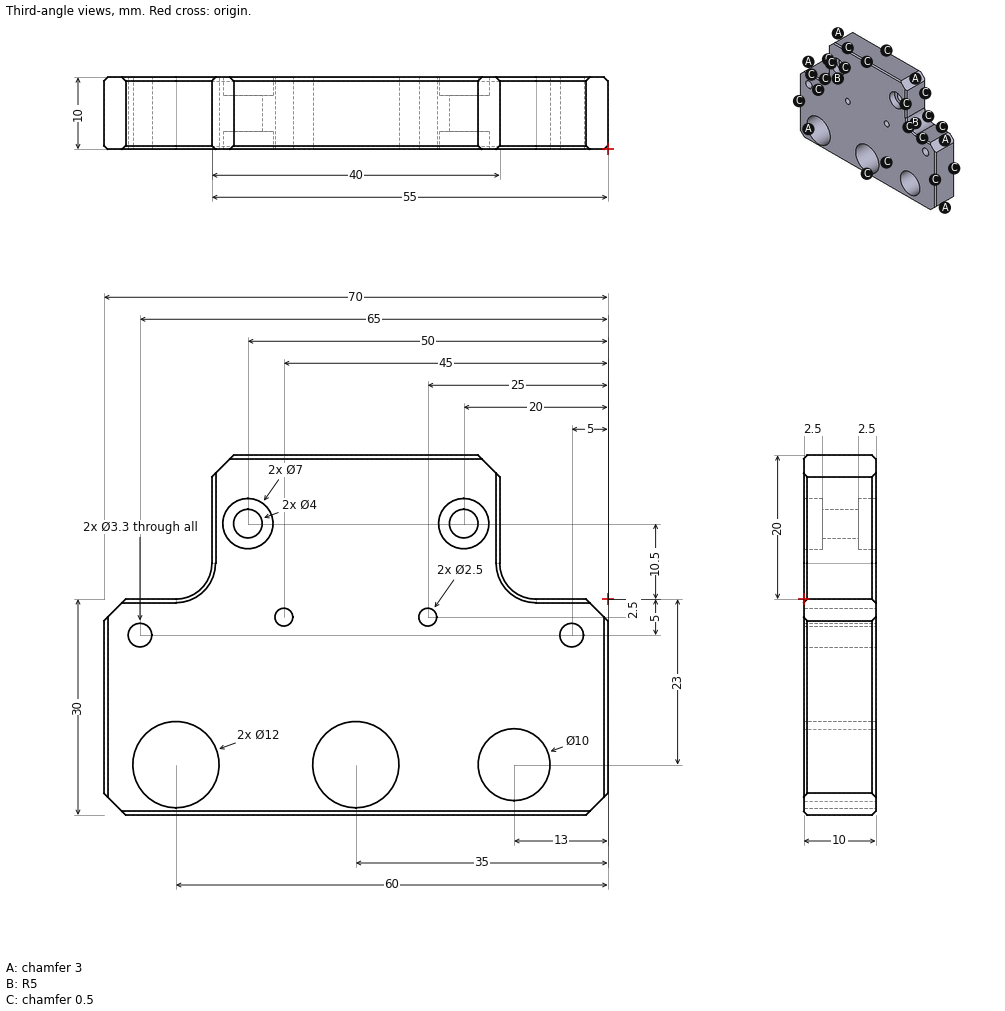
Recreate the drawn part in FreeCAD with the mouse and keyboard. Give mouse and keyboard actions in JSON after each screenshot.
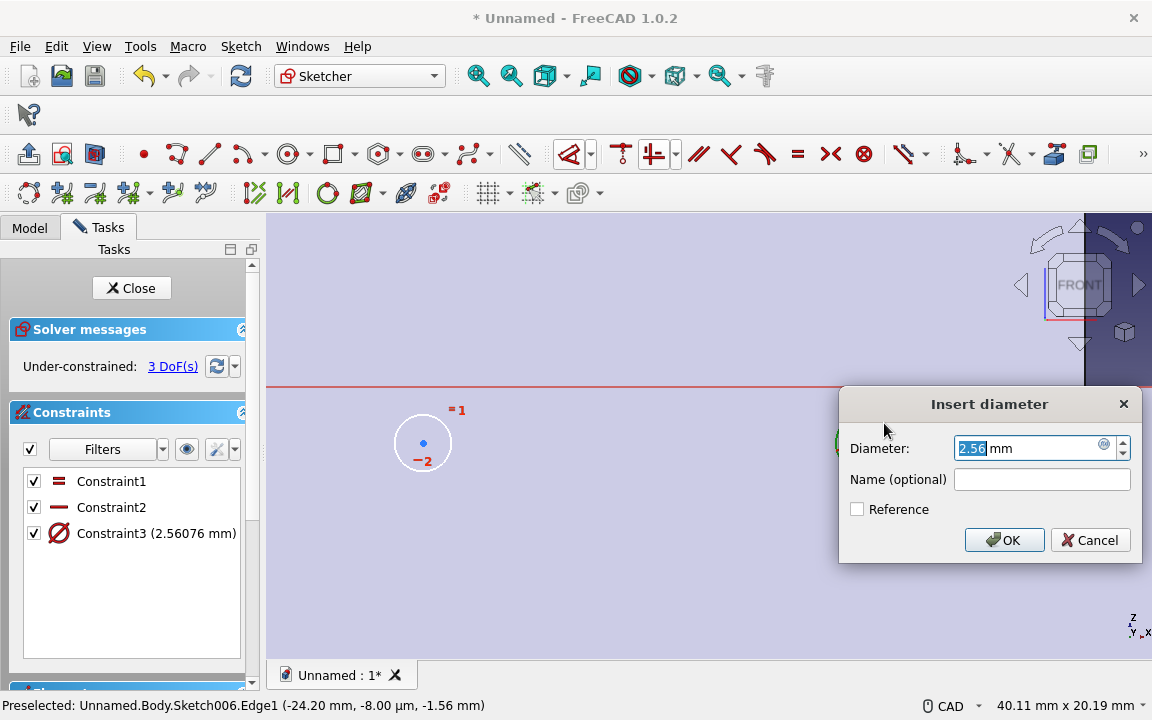
{"action": "type", "text": "2.5"}
{"action": "key", "text": "Return"}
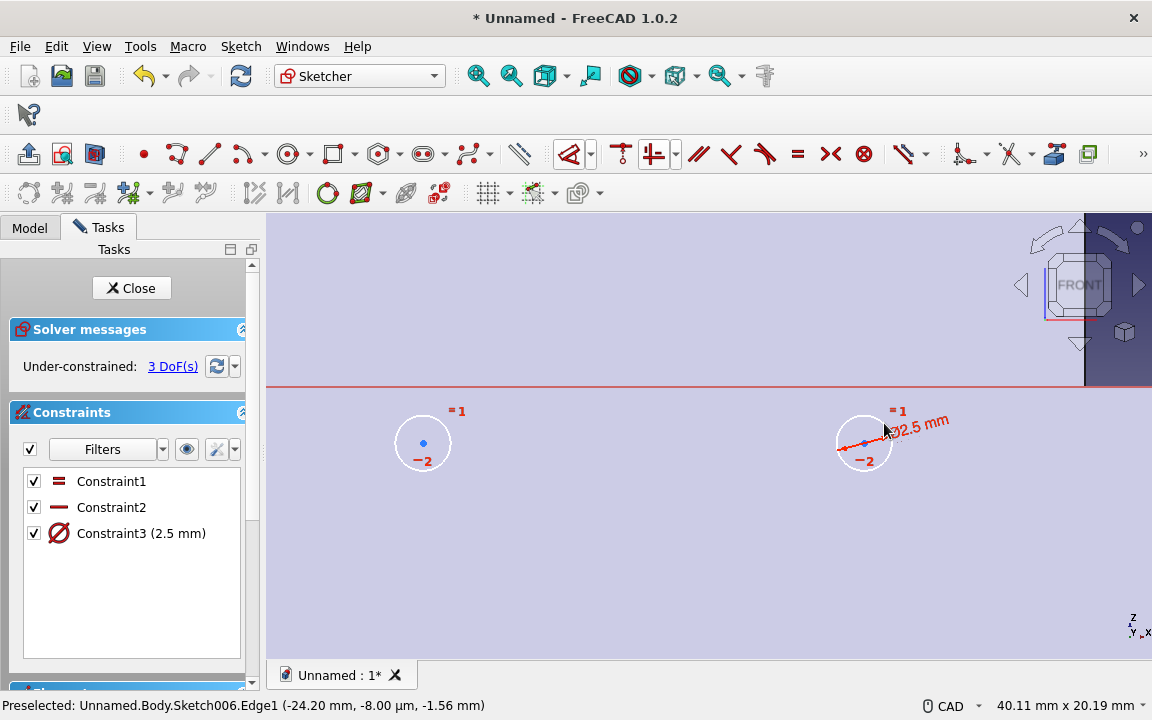
{"action": "left_click", "coordinate": [864, 443]}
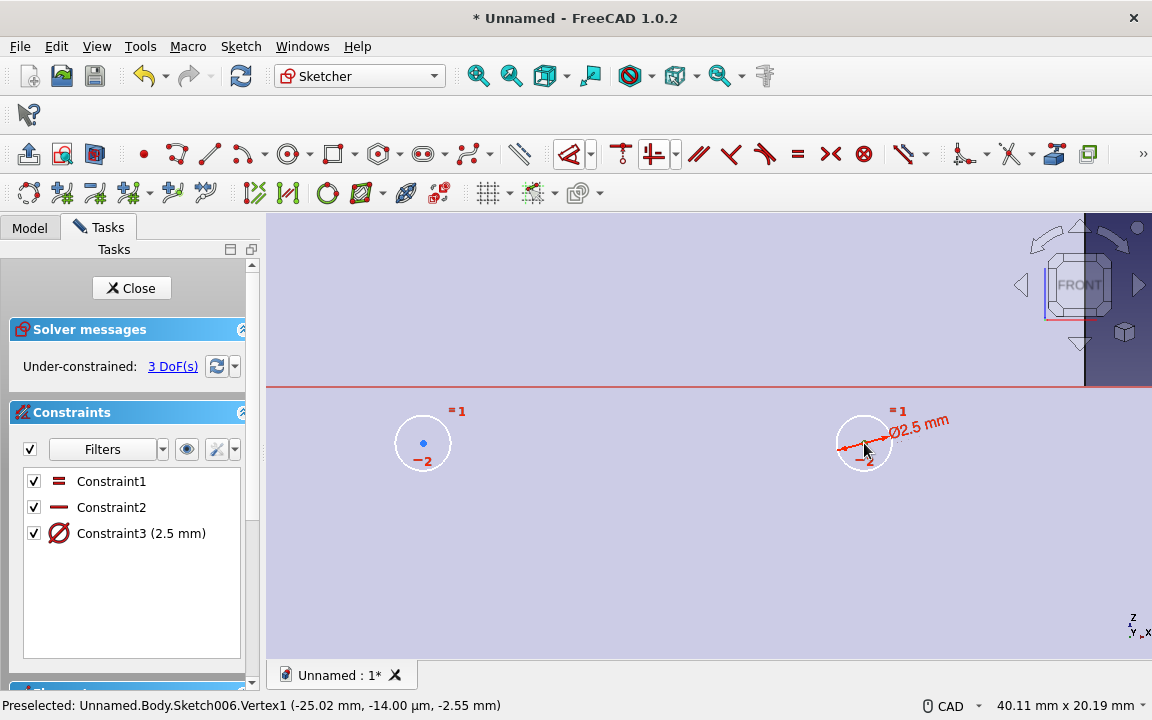
{"action": "left_click", "coordinate": [590, 154]}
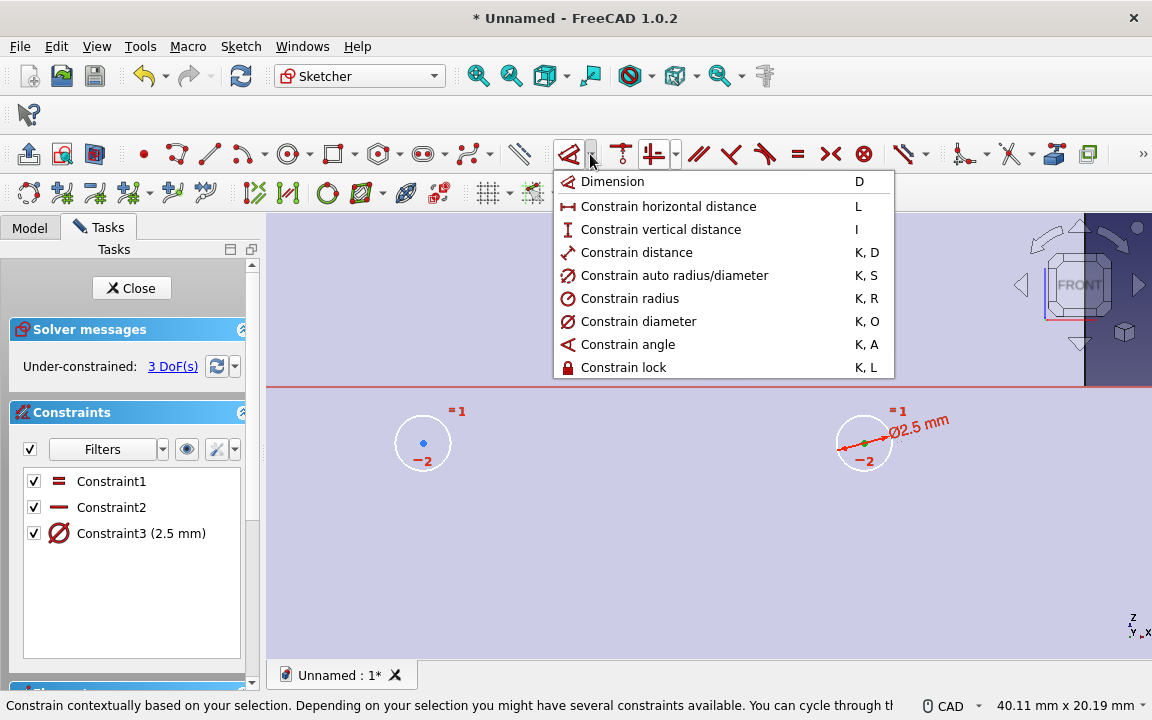
{"action": "left_click", "coordinate": [724, 206]}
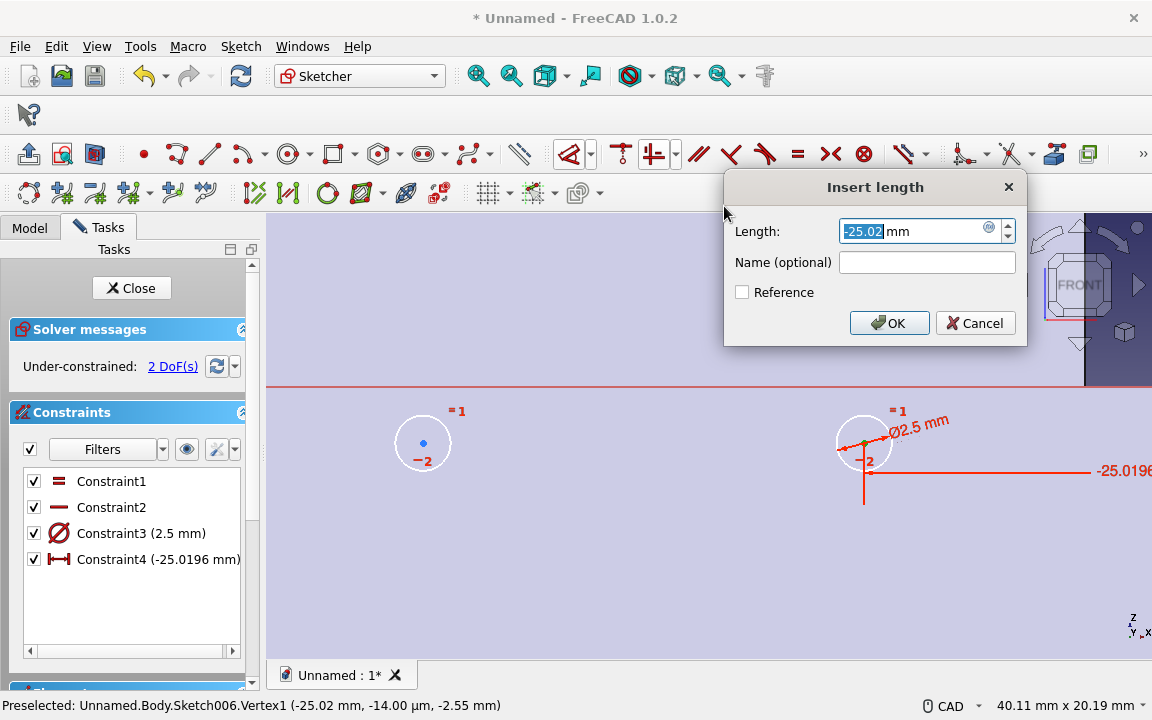
{"action": "type", "text": "-25"}
{"action": "key", "text": "Return"}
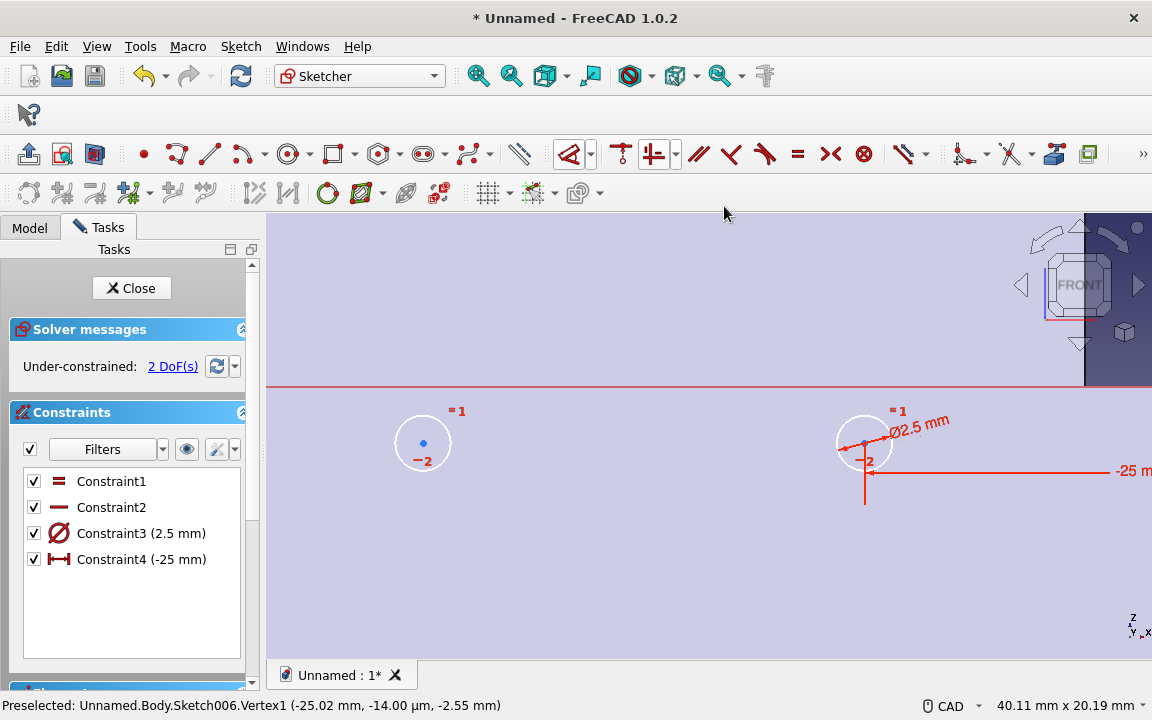
{"action": "left_click", "coordinate": [423, 443]}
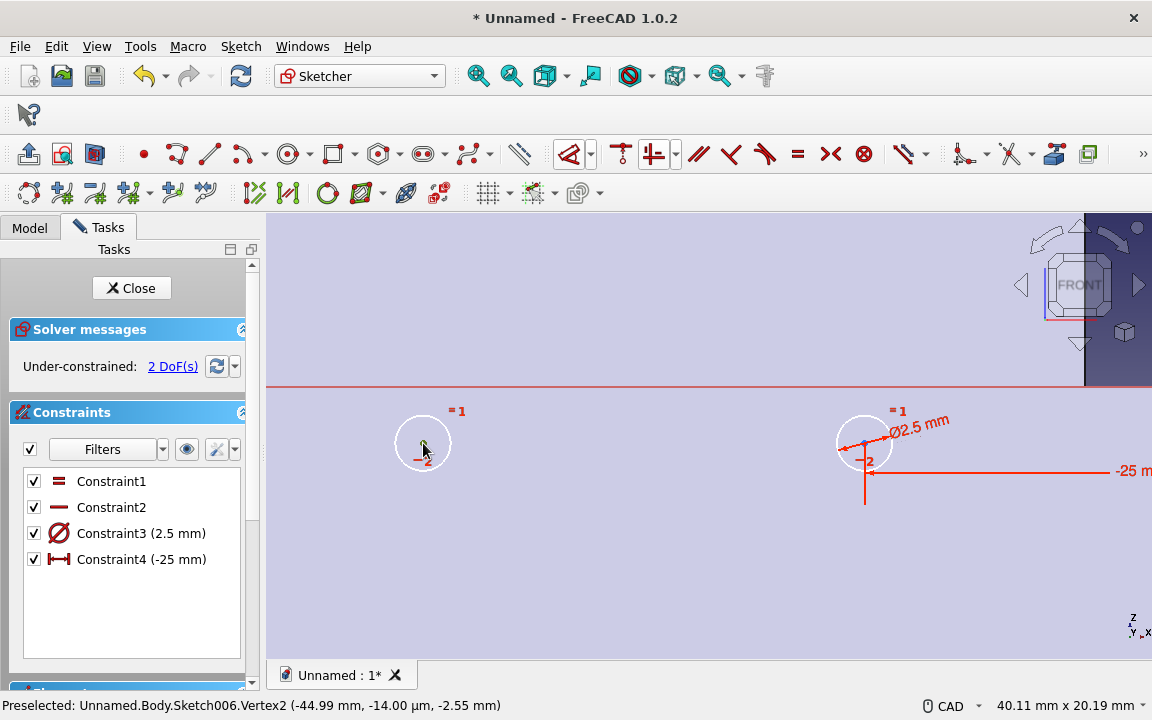
{"action": "left_click", "coordinate": [590, 154]}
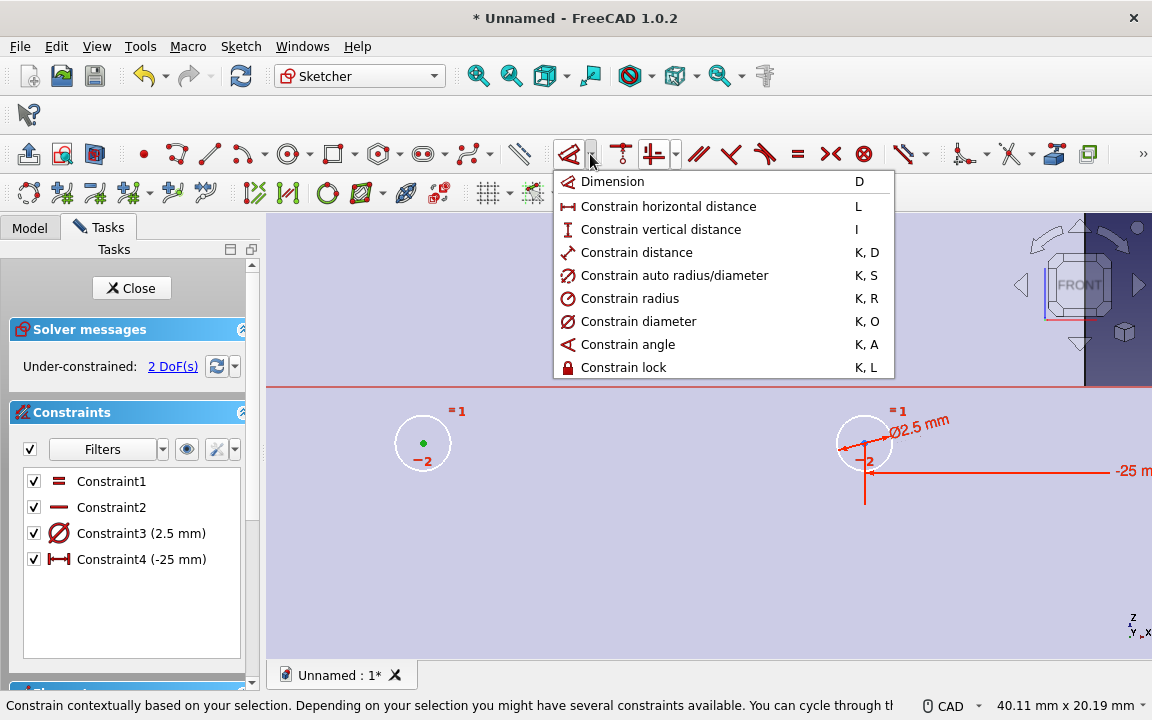
{"action": "left_click", "coordinate": [724, 206]}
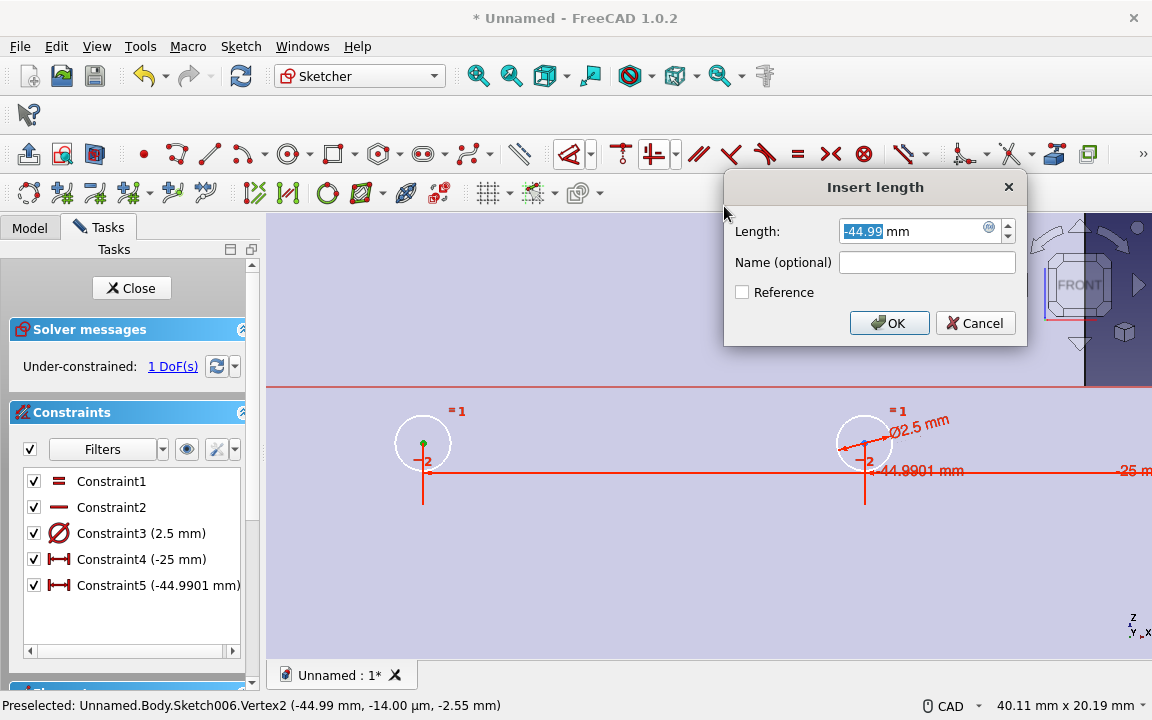
{"action": "type", "text": "-45"}
{"action": "key", "text": "Return"}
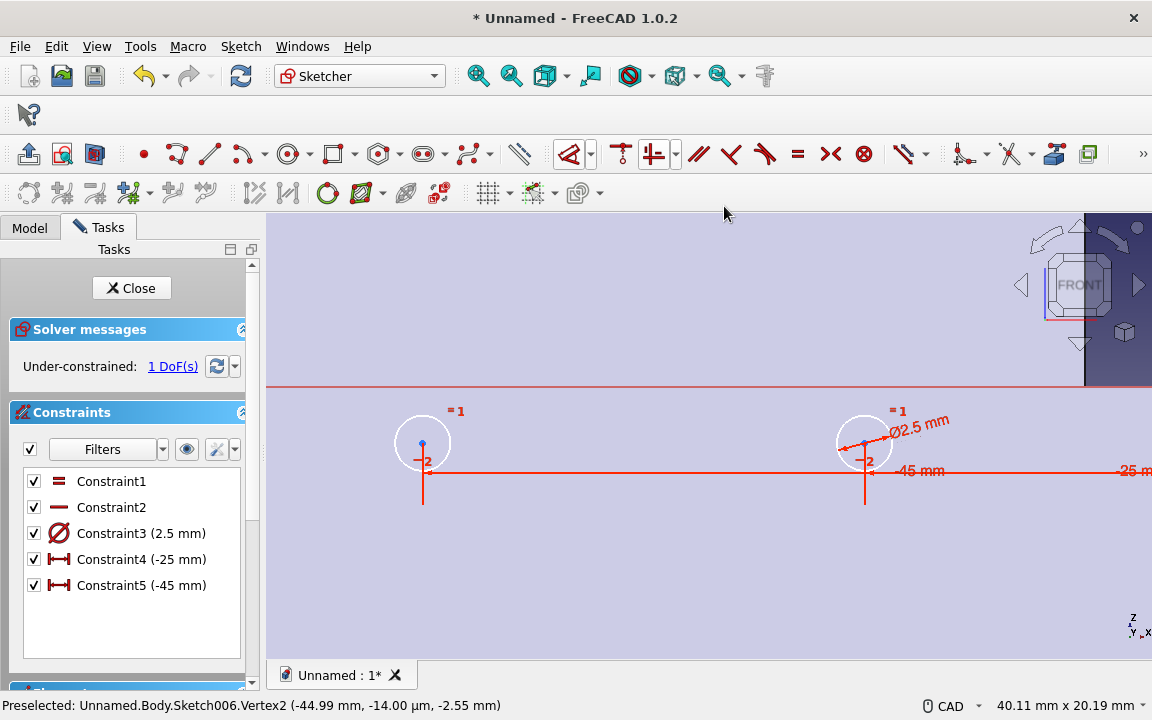
{"action": "left_click", "coordinate": [865, 443]}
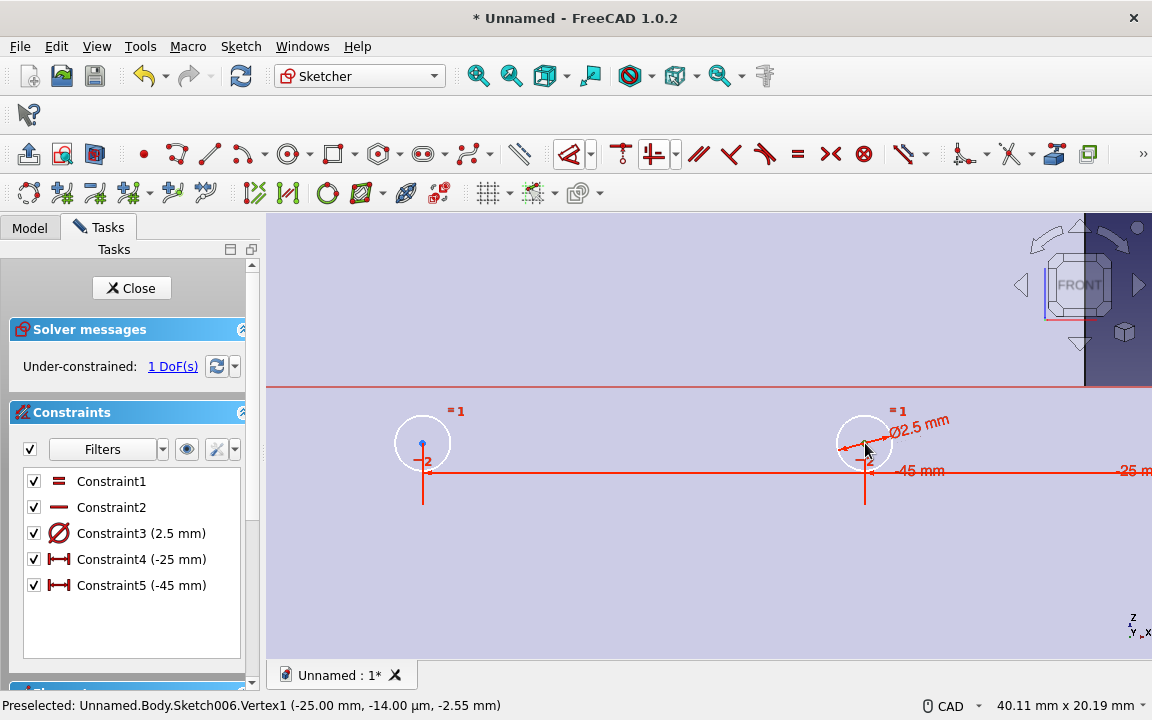
{"action": "key", "text": "i"}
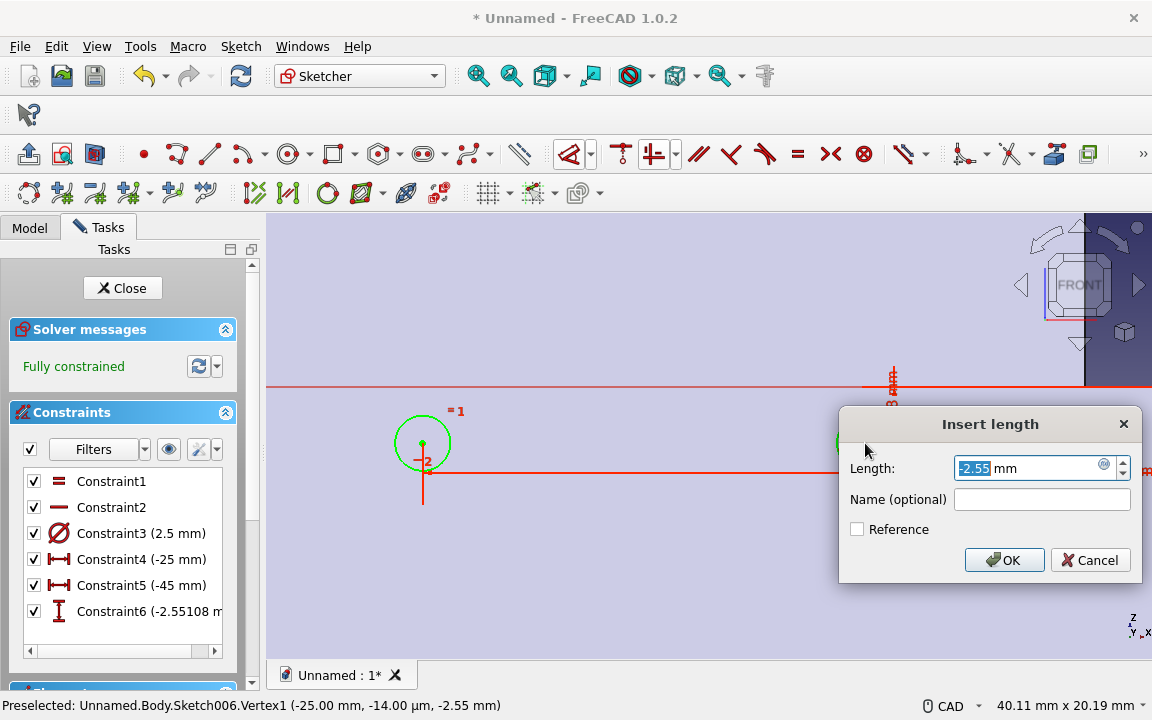
{"action": "type", "text": "-2.5"}
{"action": "key", "text": "Return"}